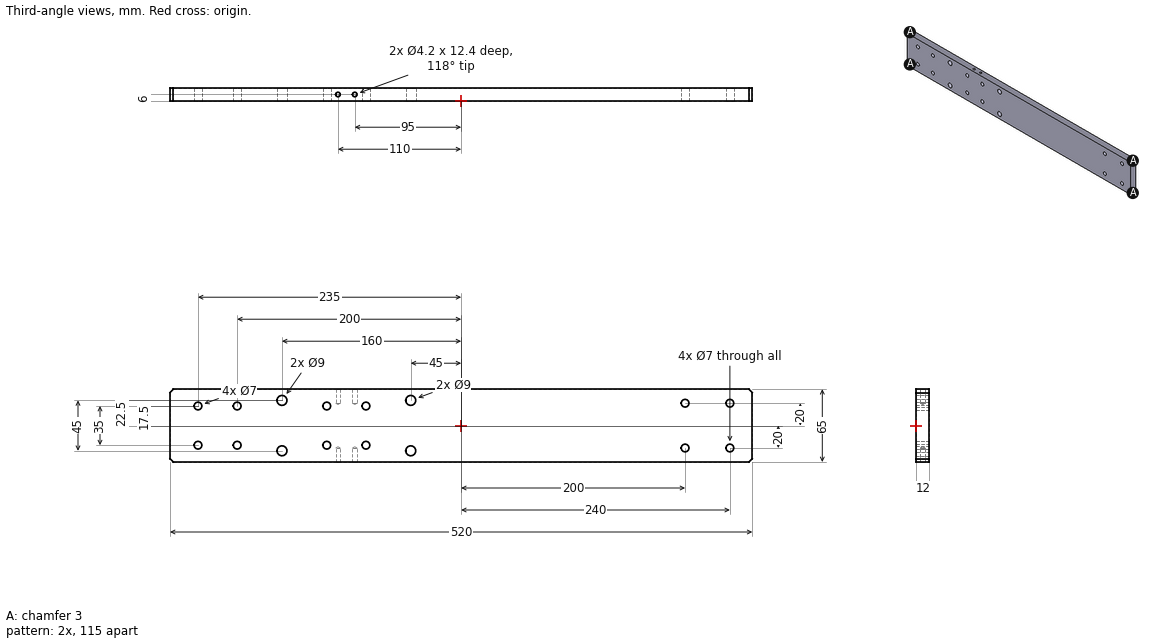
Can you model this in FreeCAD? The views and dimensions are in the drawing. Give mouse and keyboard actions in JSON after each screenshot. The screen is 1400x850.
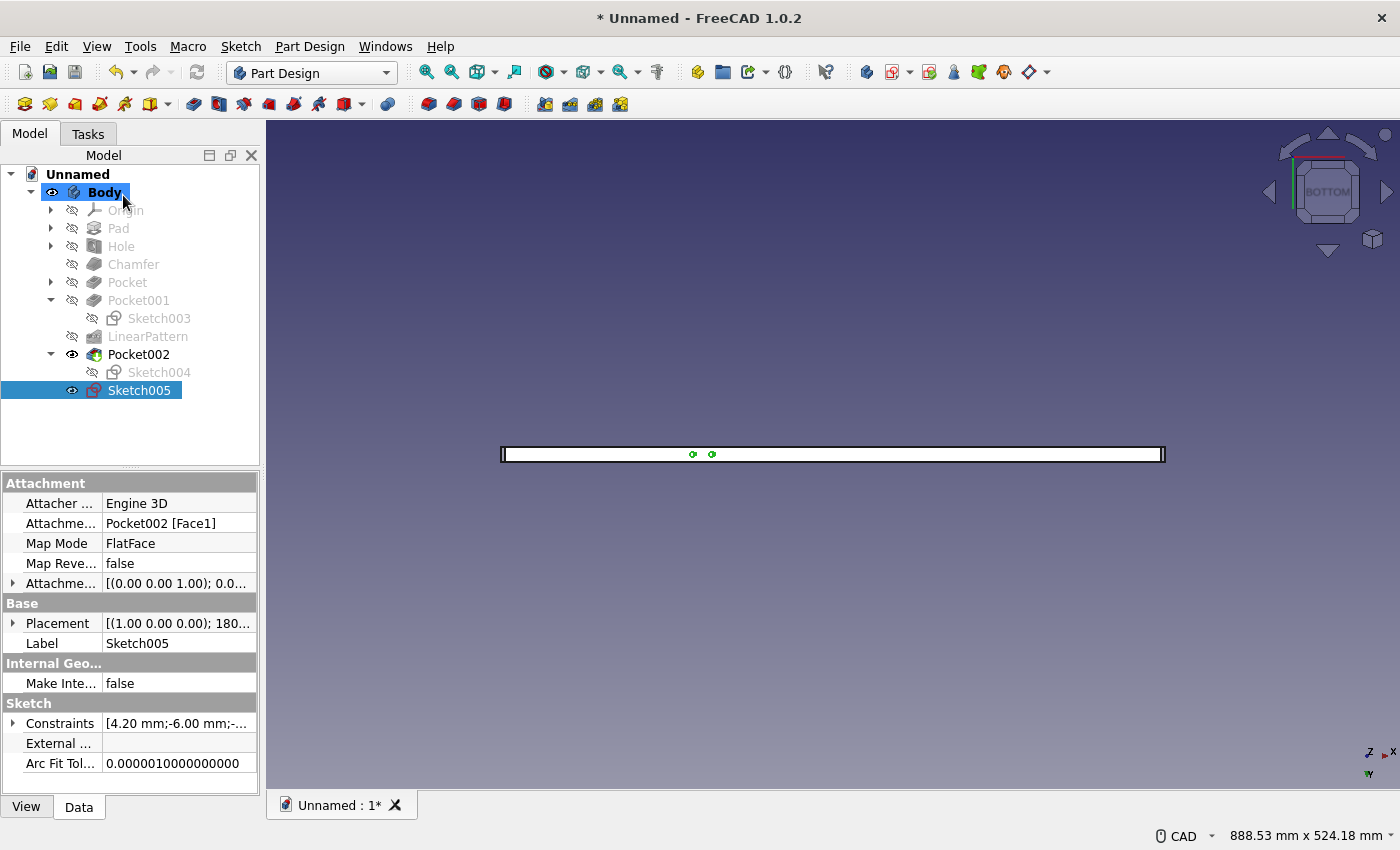
{"action": "left_click", "coordinate": [219, 104]}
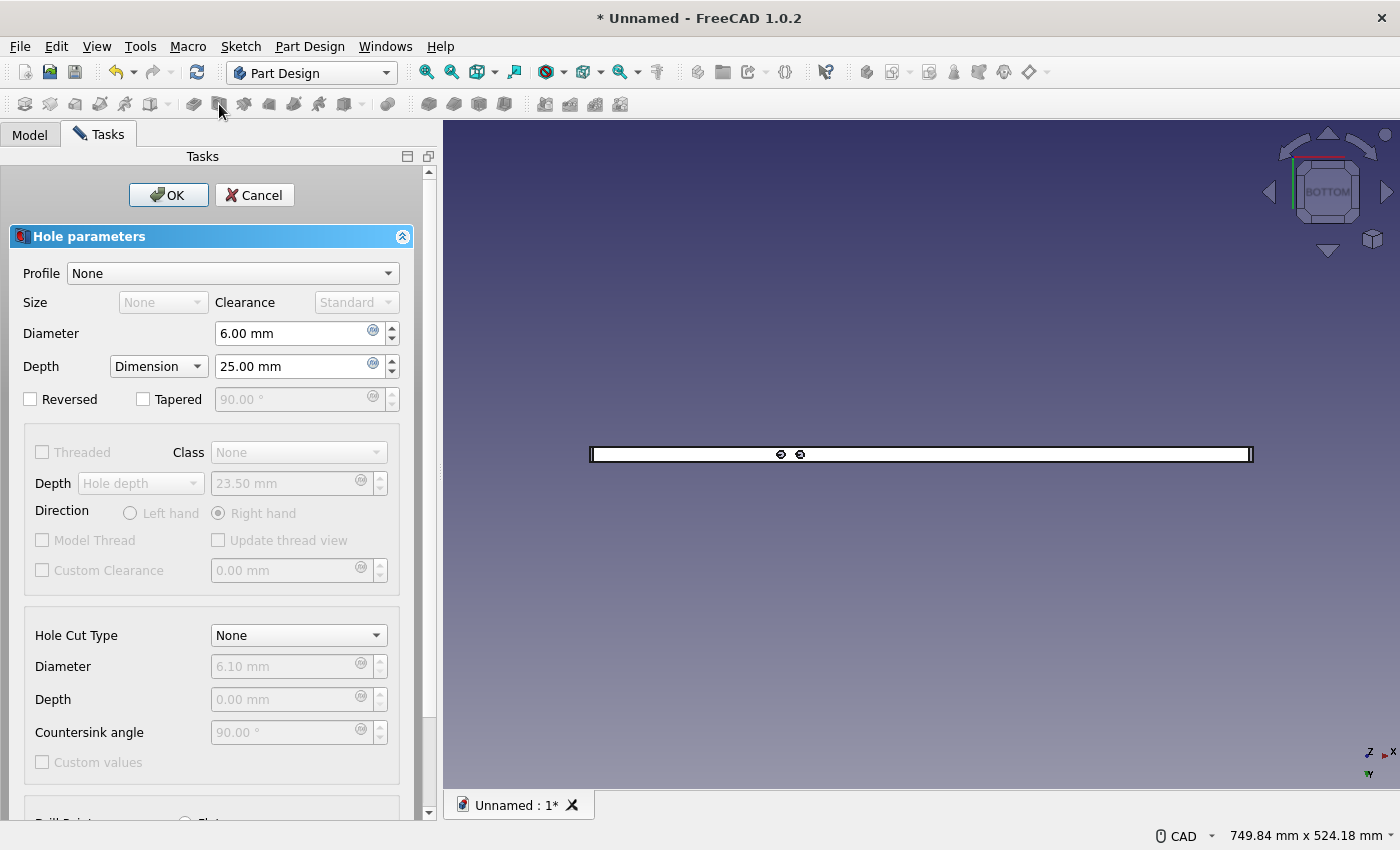
{"action": "triple_click", "coordinate": [300, 334]}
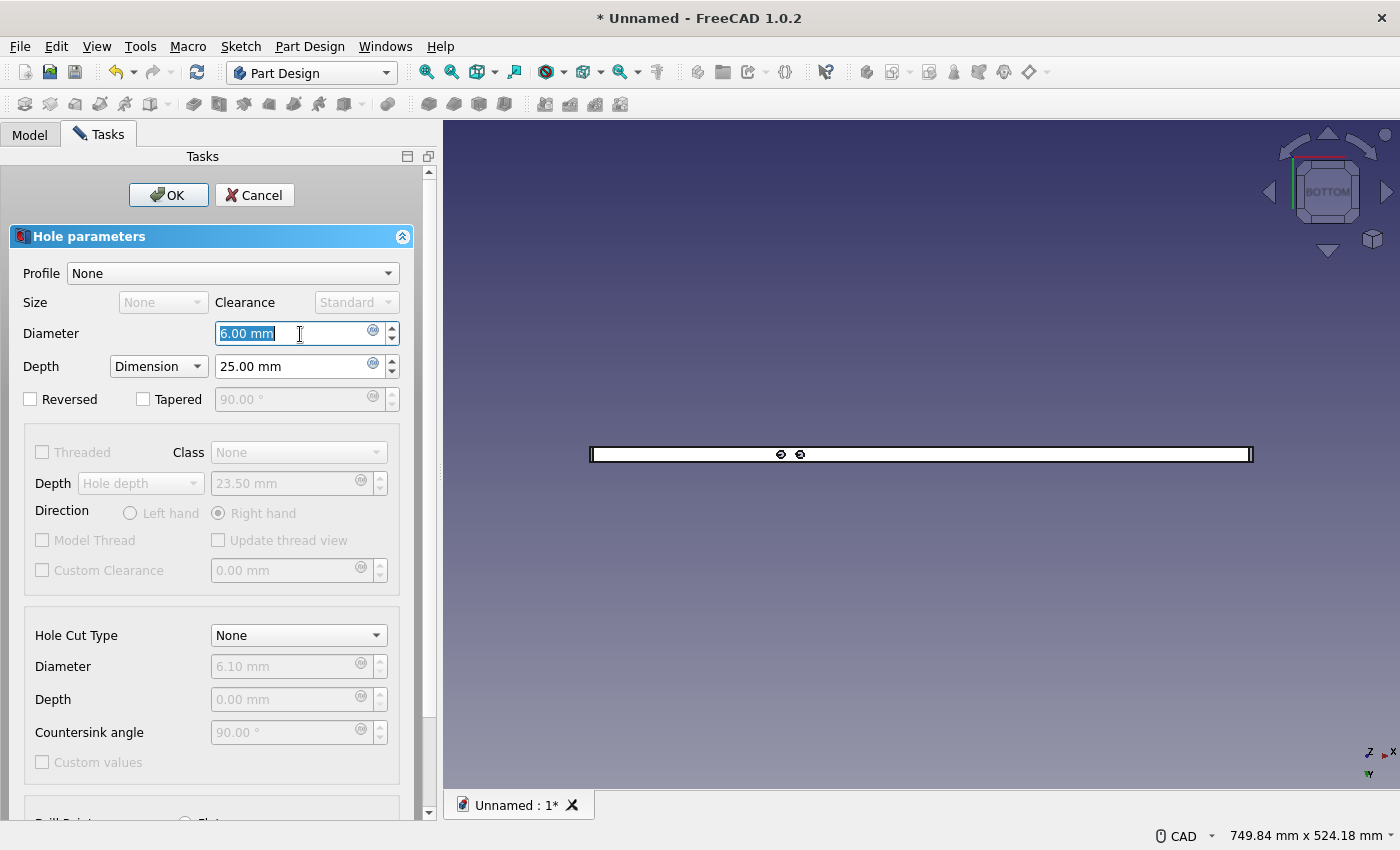
{"action": "type", "text": "4.2"}
{"action": "key", "text": "Tab"}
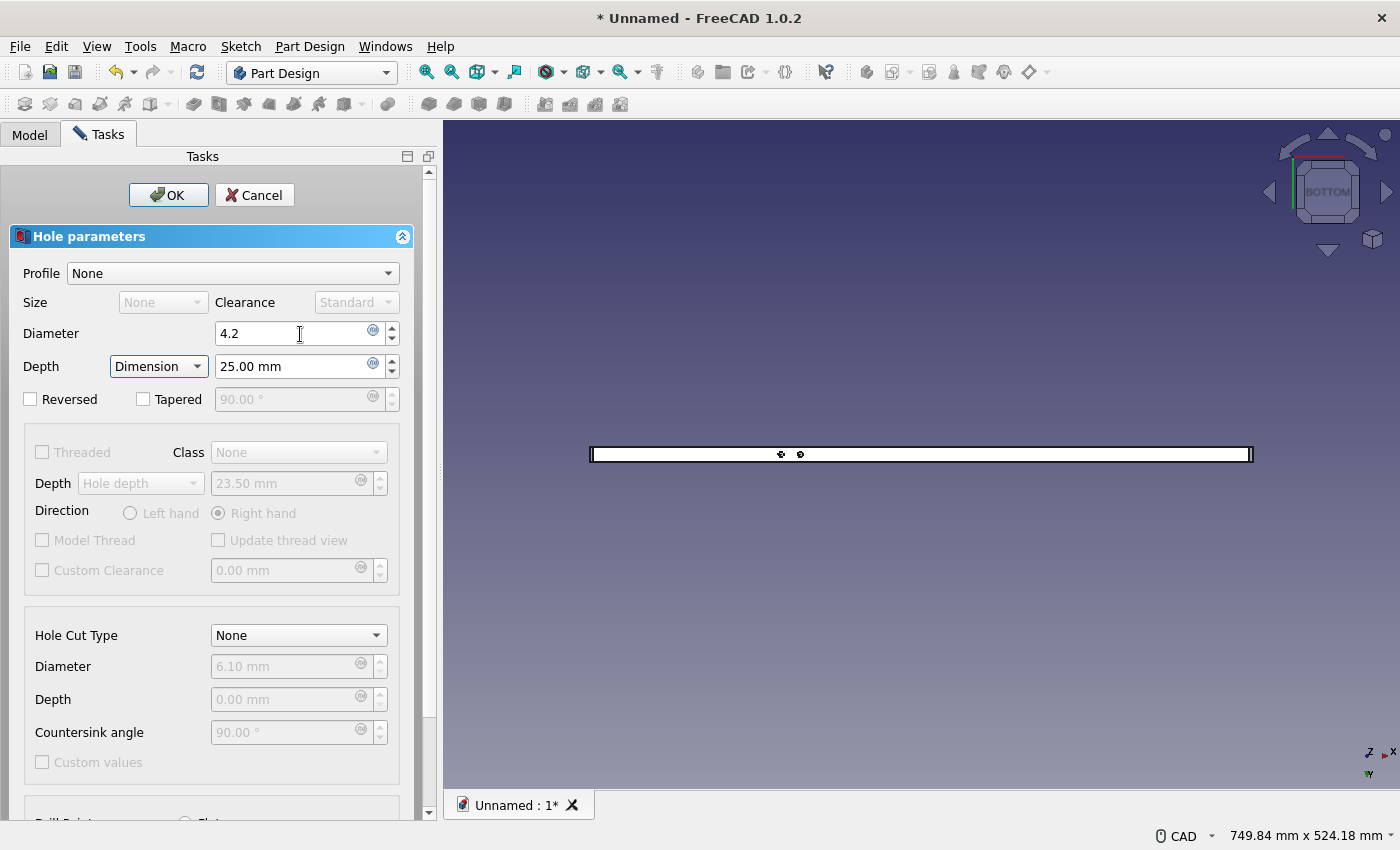
{"action": "triple_click", "coordinate": [300, 366]}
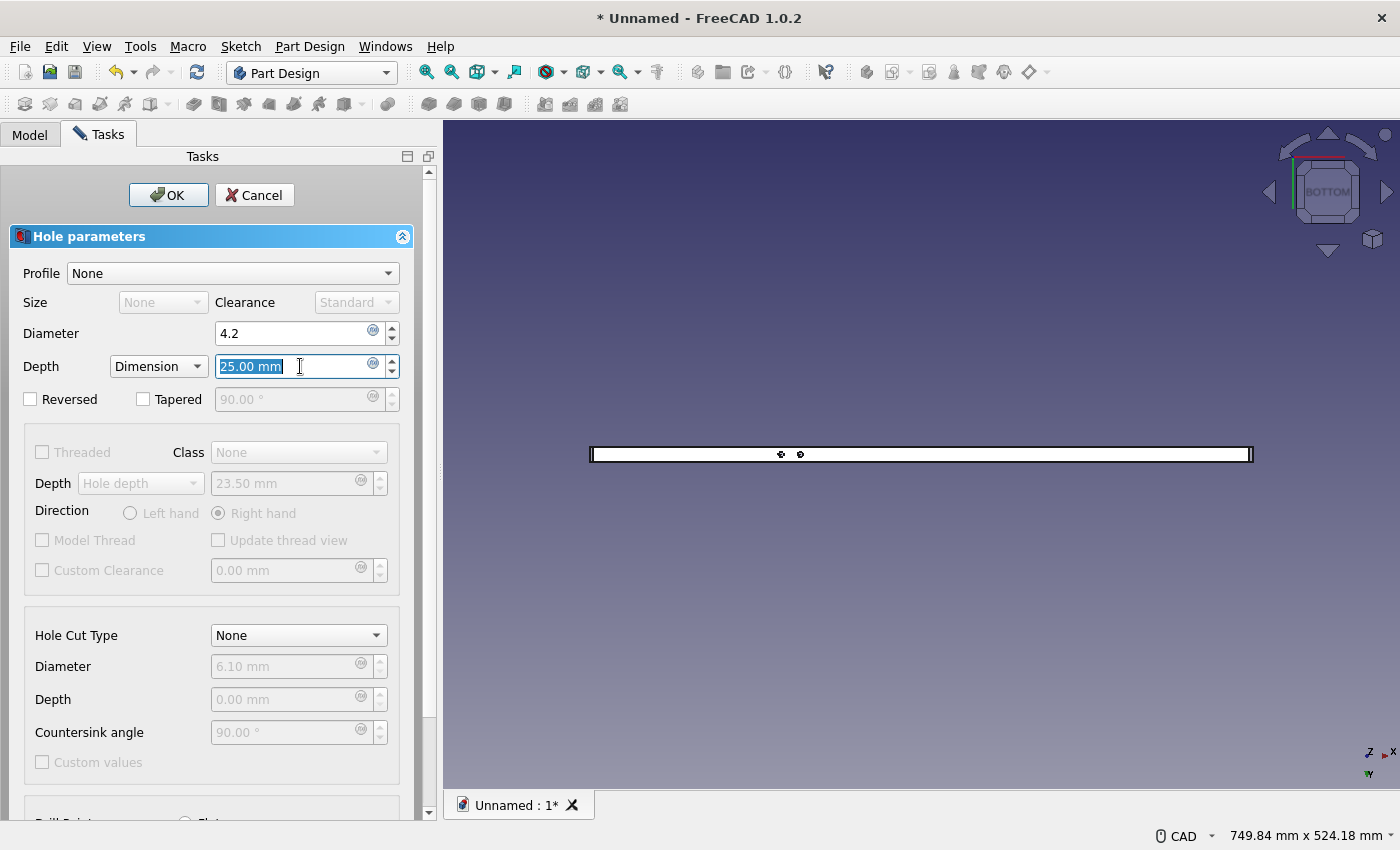
{"action": "type", "text": "12.4"}
{"action": "key", "text": "Tab"}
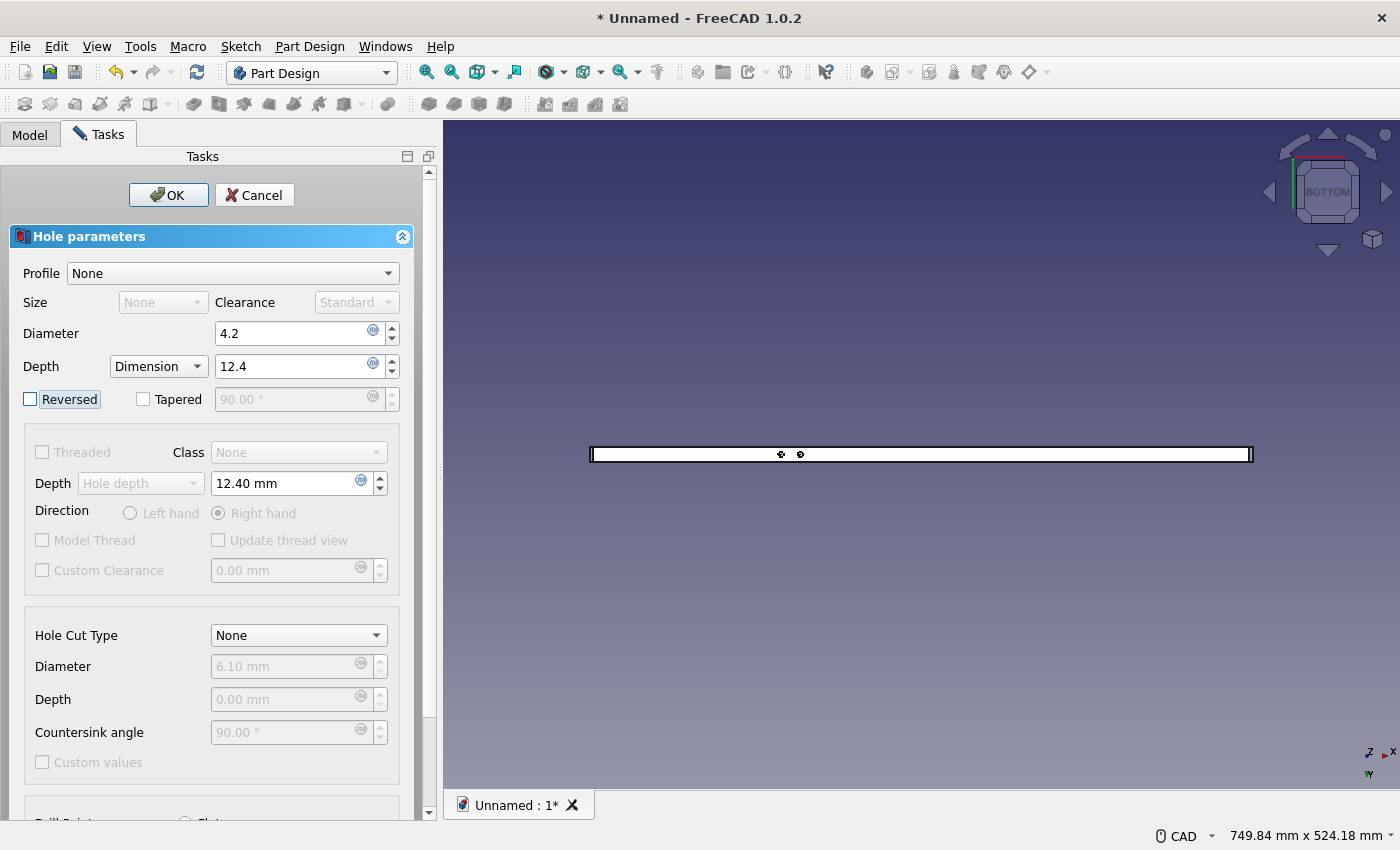
{"action": "left_click", "coordinate": [169, 195]}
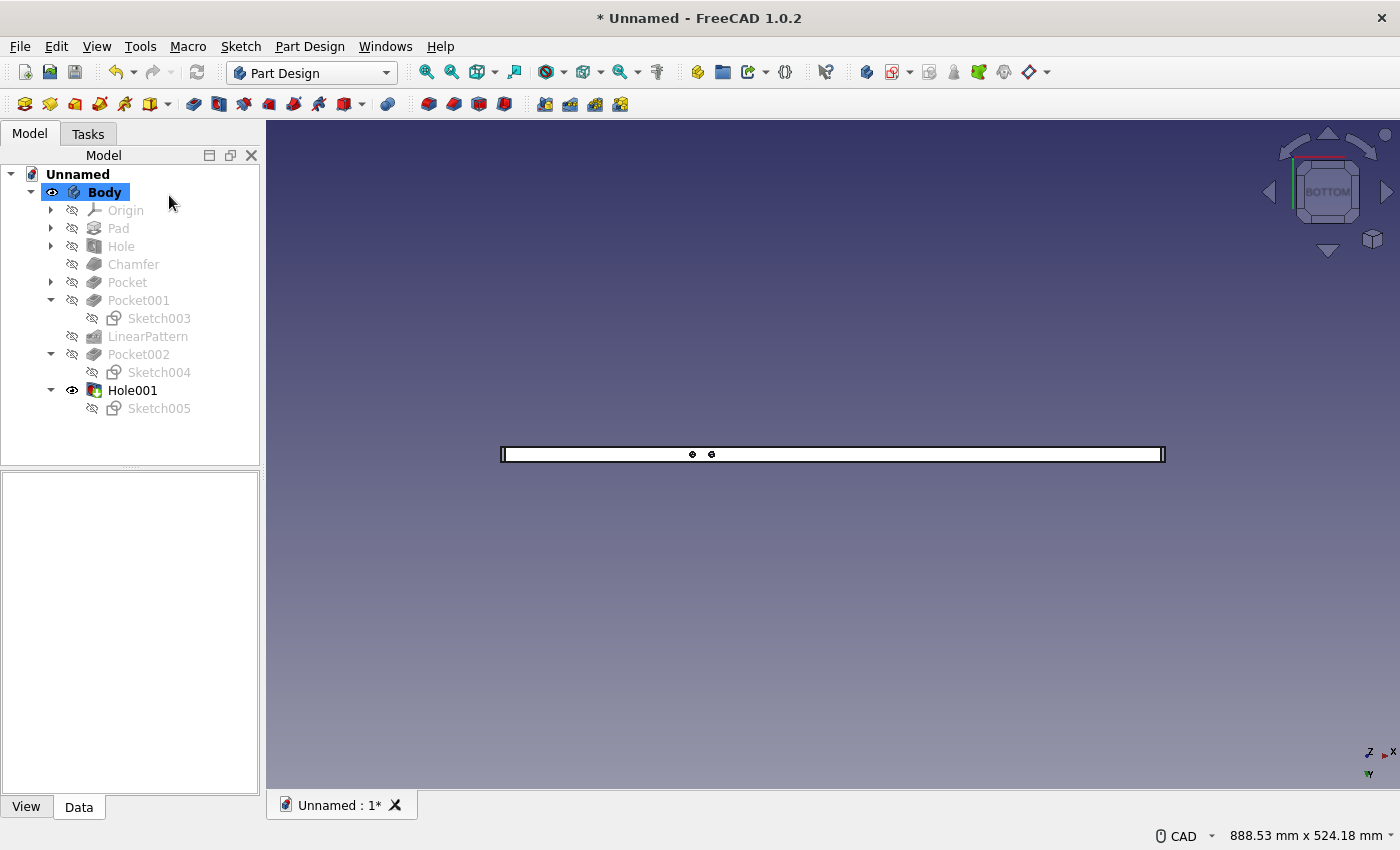
{"action": "key", "text": "0"}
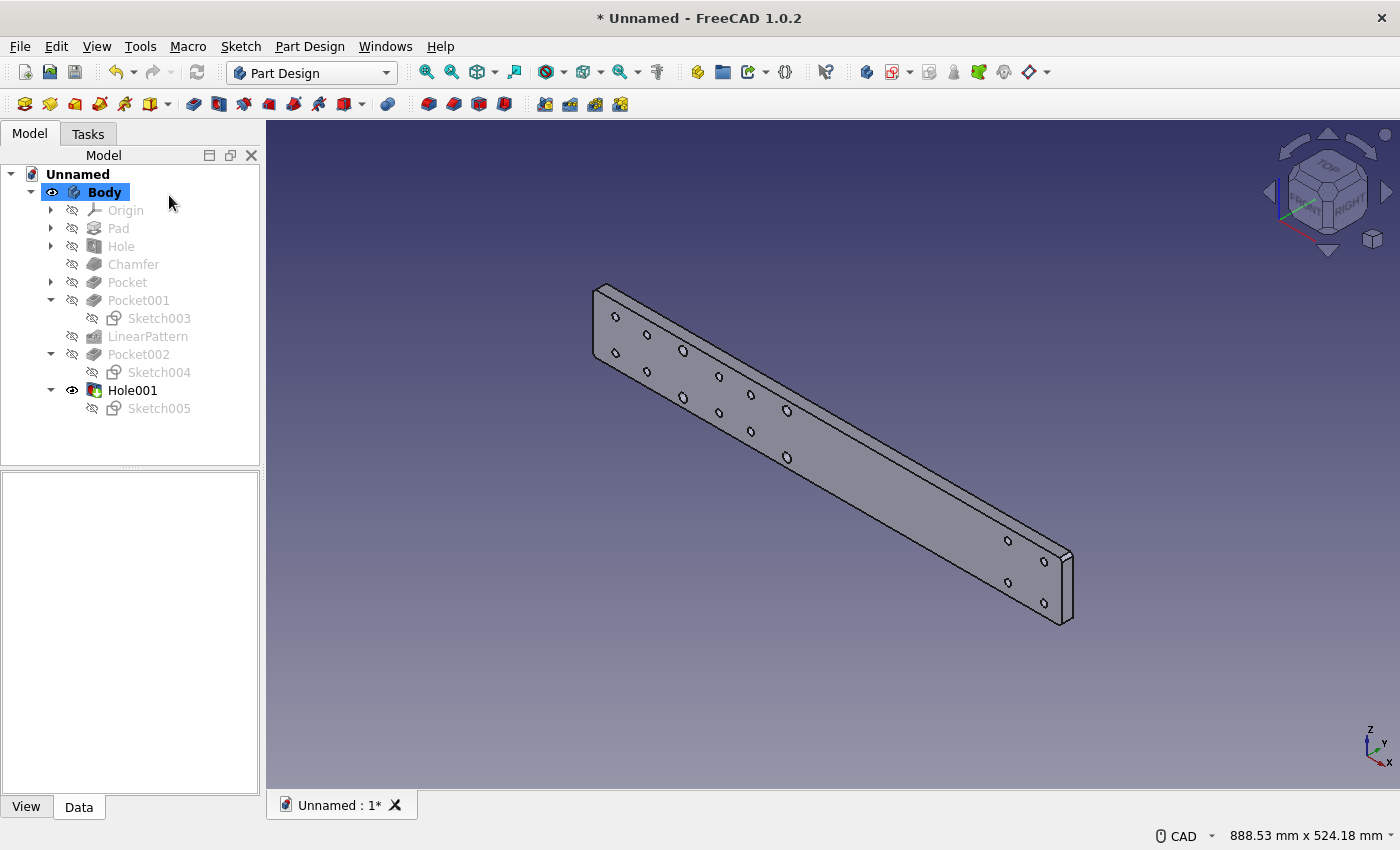
{"action": "key", "text": "2"}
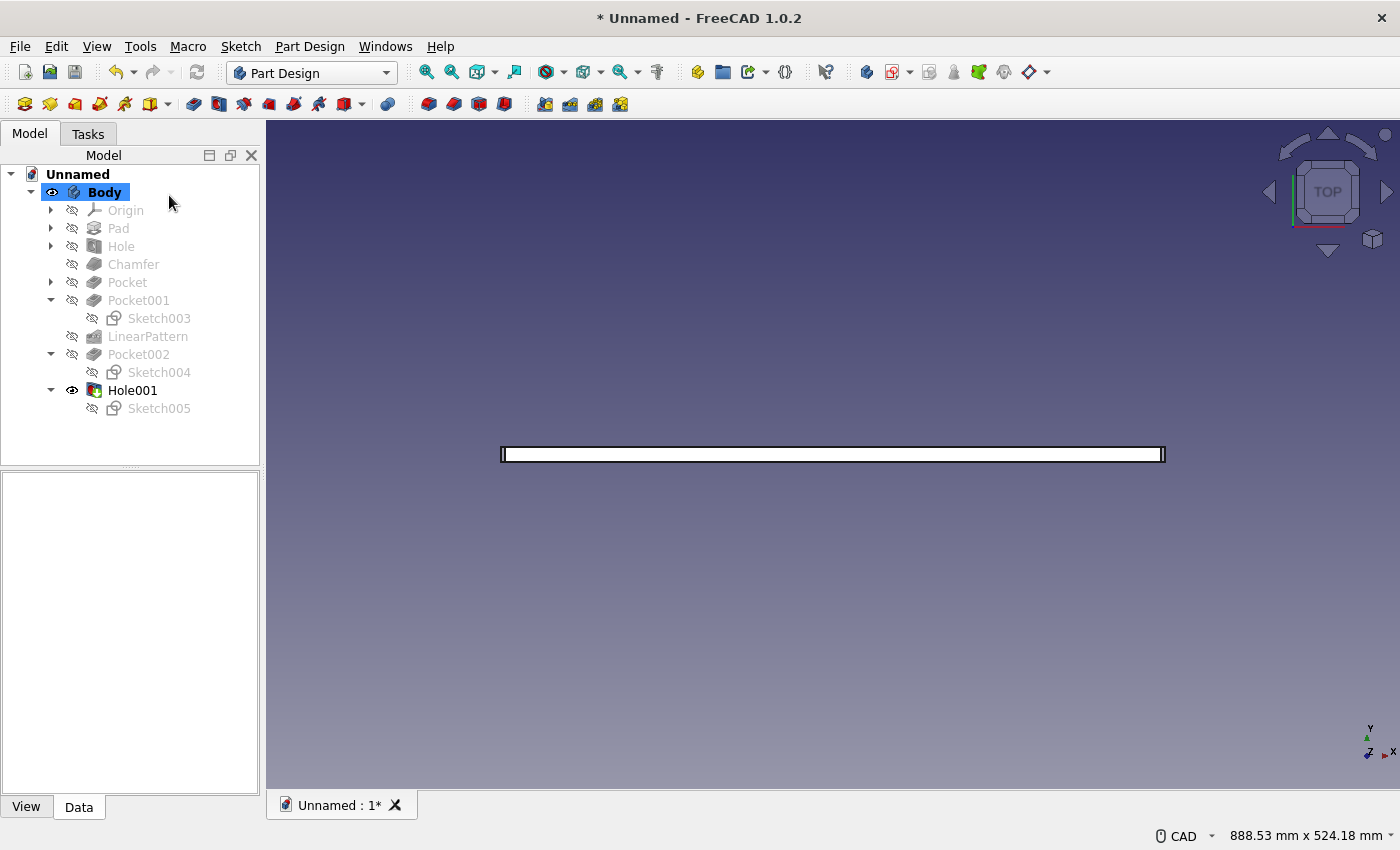
{"action": "key", "text": "4"}